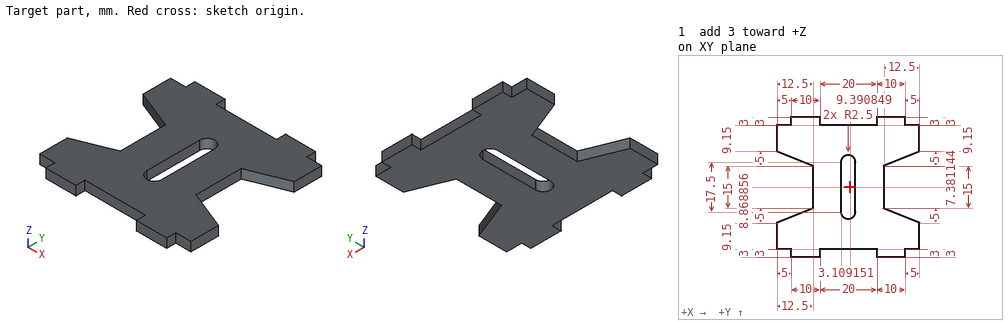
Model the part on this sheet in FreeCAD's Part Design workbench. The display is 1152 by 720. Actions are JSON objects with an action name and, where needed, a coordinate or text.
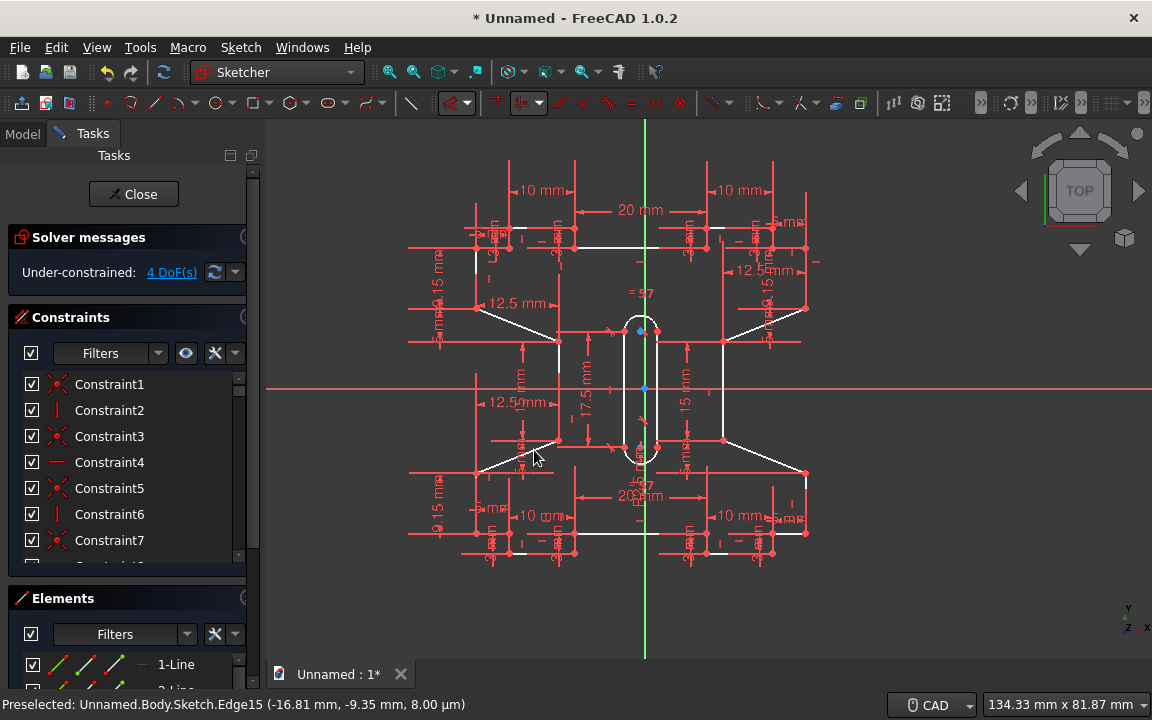
{"action": "left_click", "coordinate": [723, 342]}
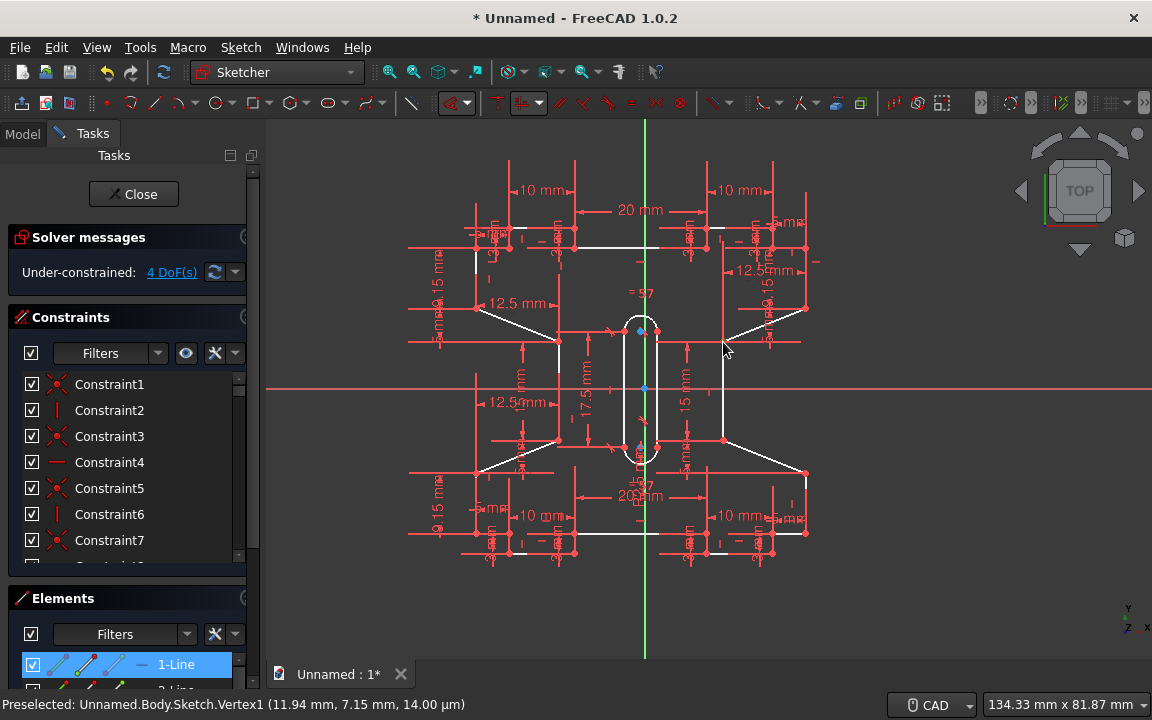
{"action": "left_click", "coordinate": [470, 104]}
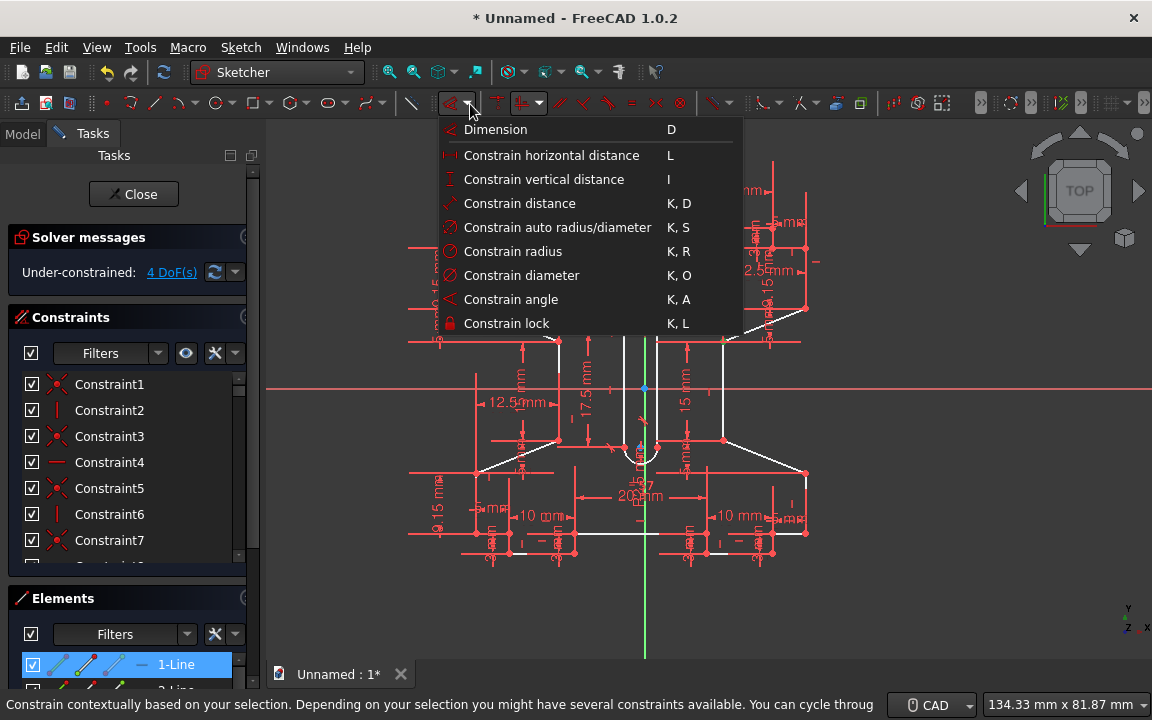
{"action": "left_click", "coordinate": [591, 179]}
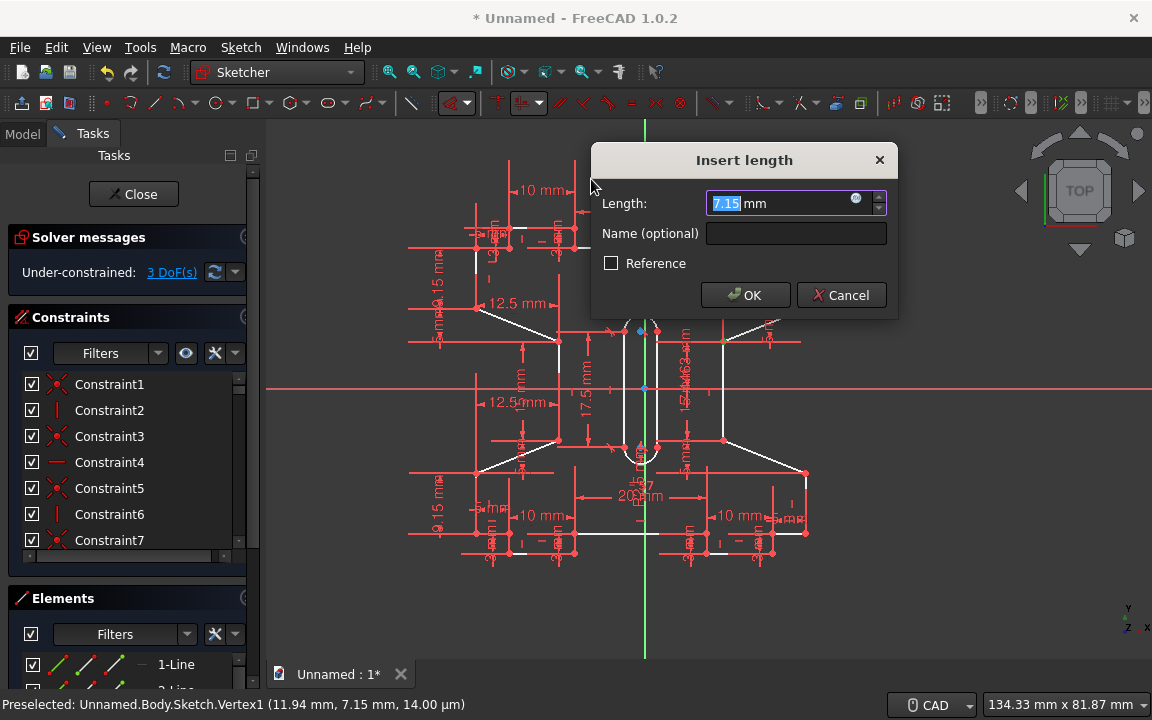
{"action": "type", "text": "7.381144"}
{"action": "key", "text": "Return"}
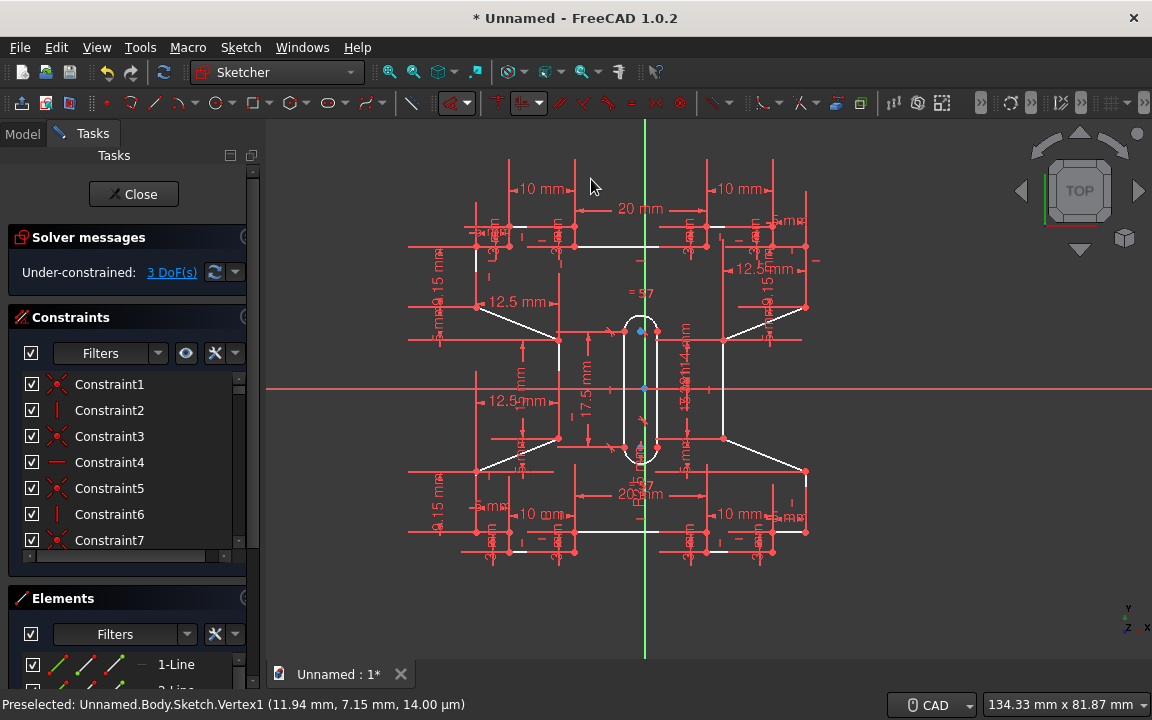
{"action": "left_click", "coordinate": [707, 227]}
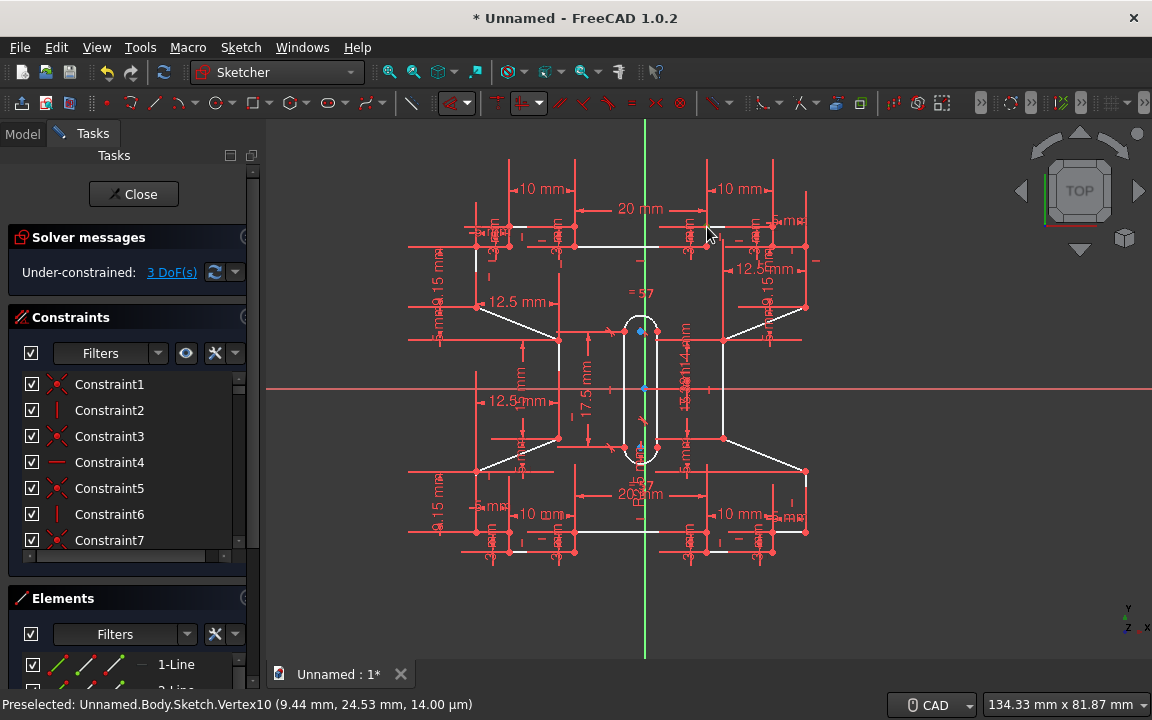
{"action": "key", "text": "l"}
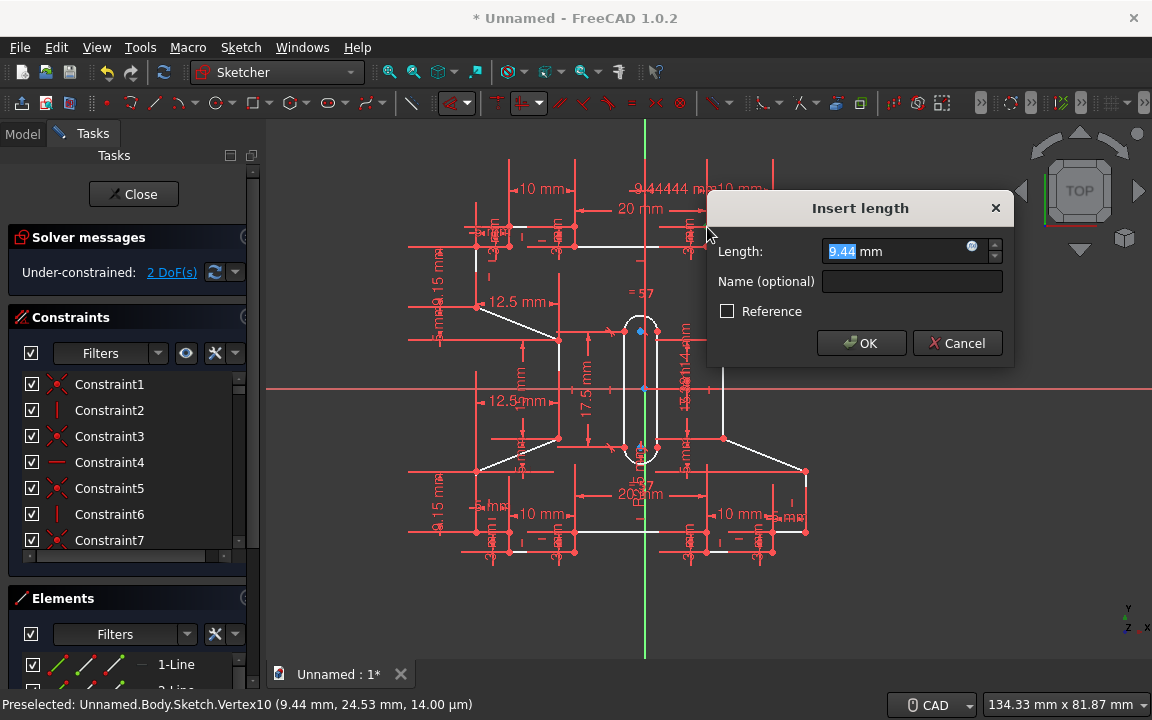
{"action": "type", "text": "9.390849"}
{"action": "key", "text": "Return"}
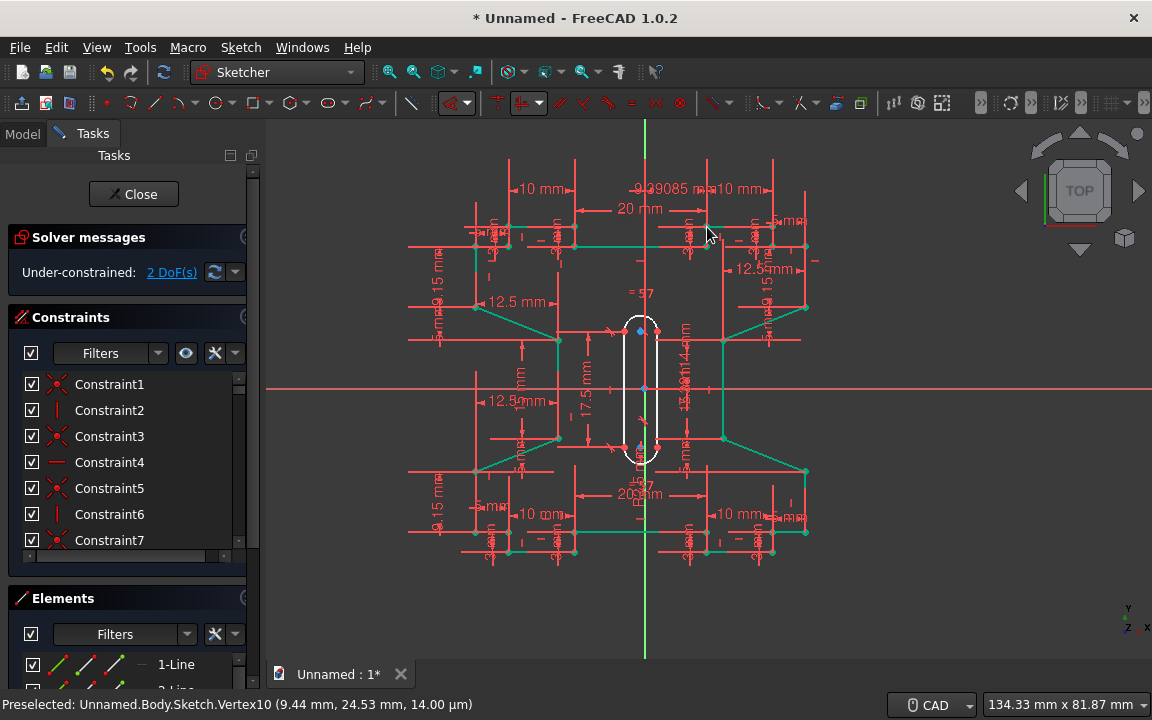
{"action": "scroll", "coordinate": [624, 447], "scroll_direction": "up", "scroll_amount": 4}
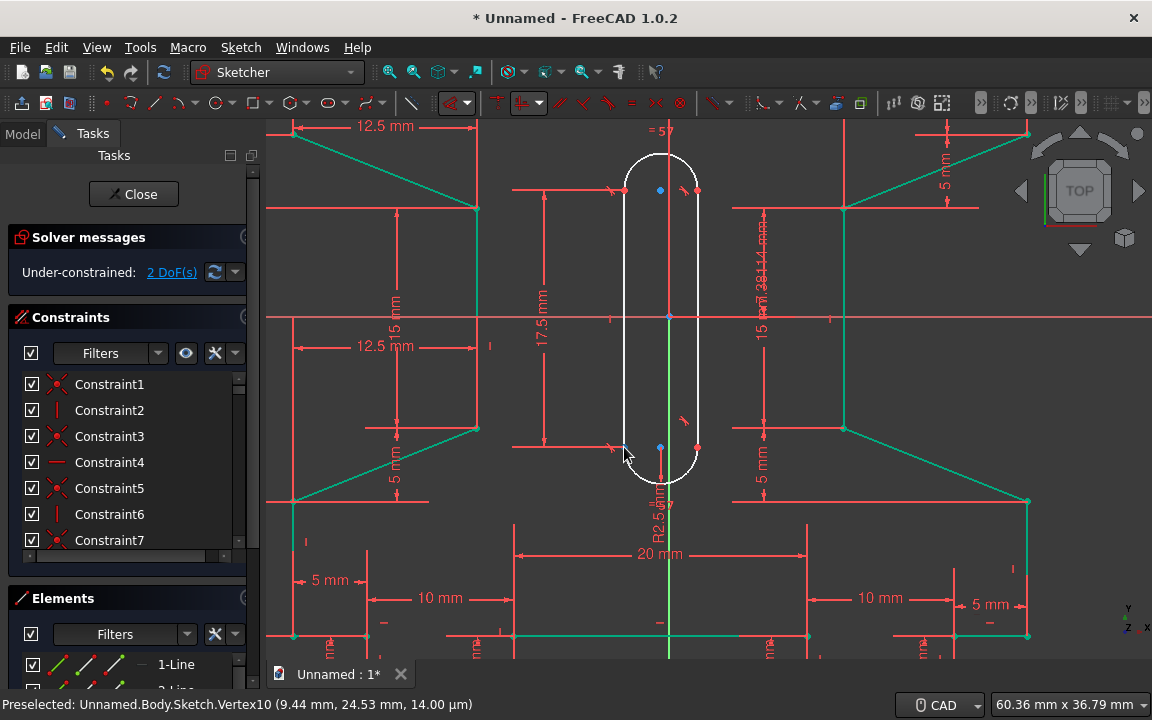
{"action": "left_click", "coordinate": [624, 447]}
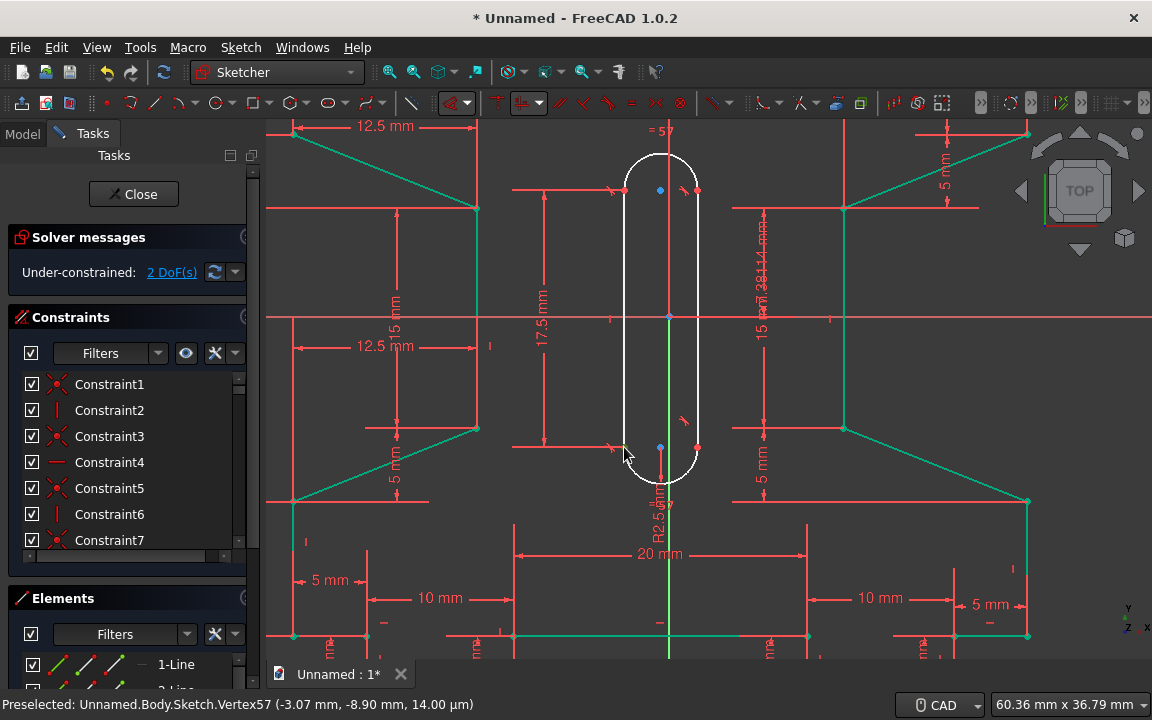
{"action": "left_click", "coordinate": [470, 104]}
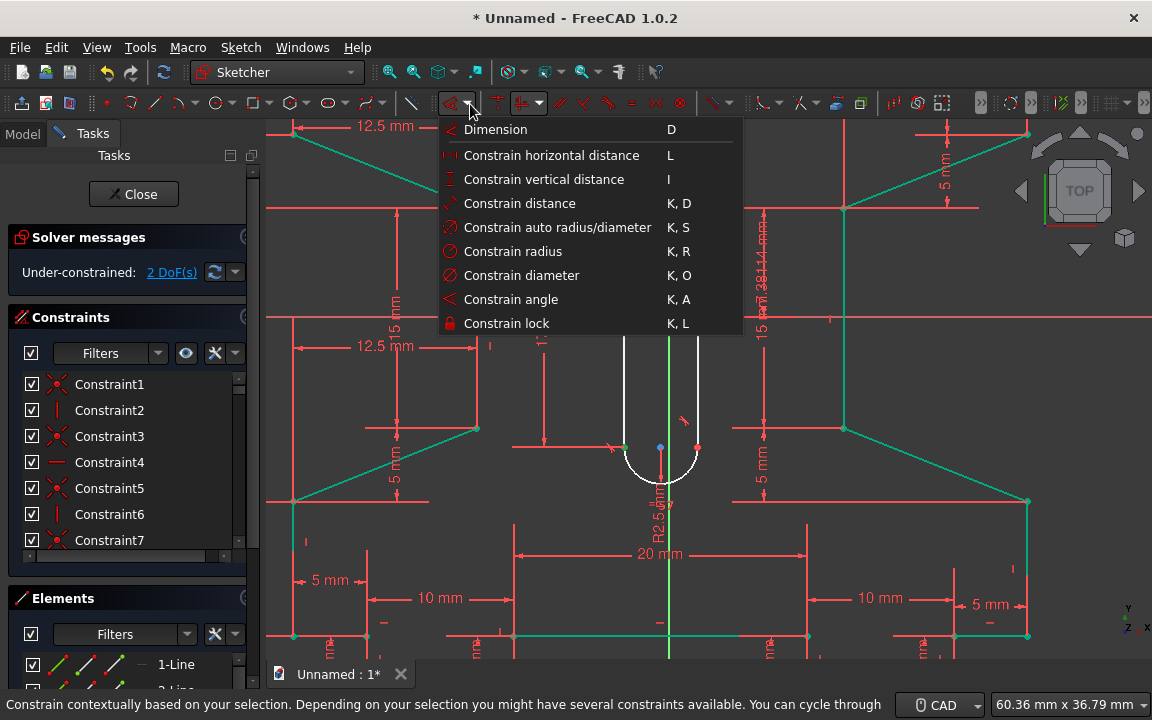
{"action": "left_click", "coordinate": [591, 155]}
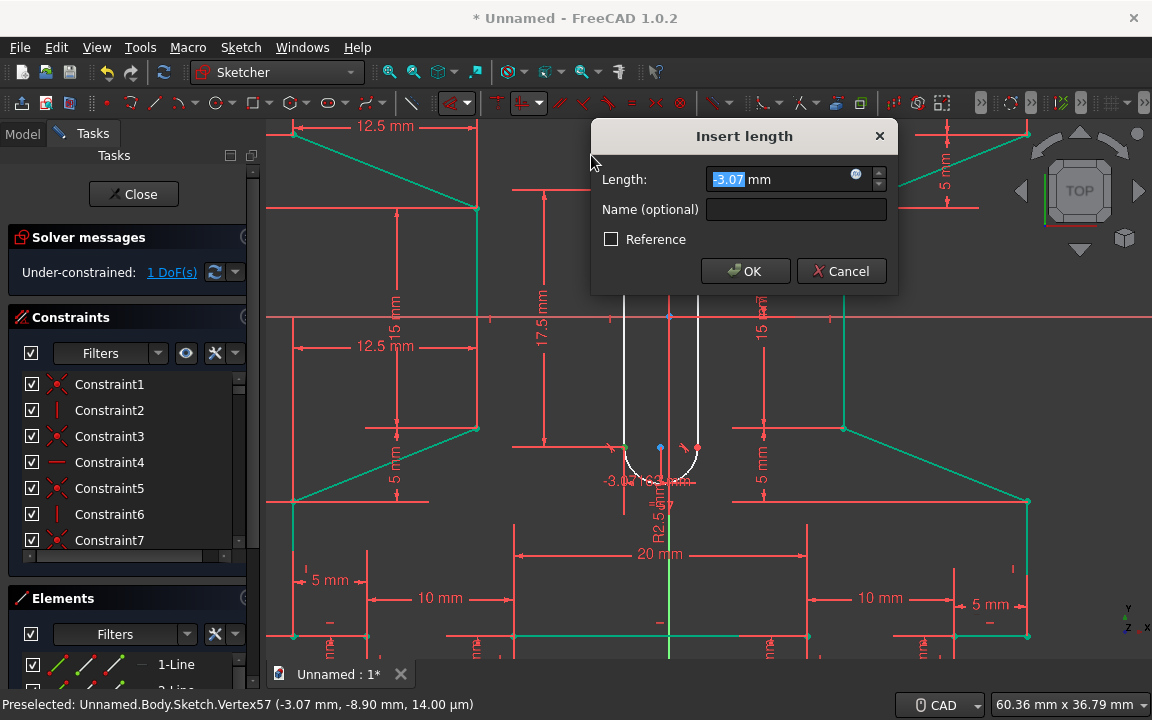
{"action": "type", "text": "-3.109151"}
{"action": "key", "text": "Return"}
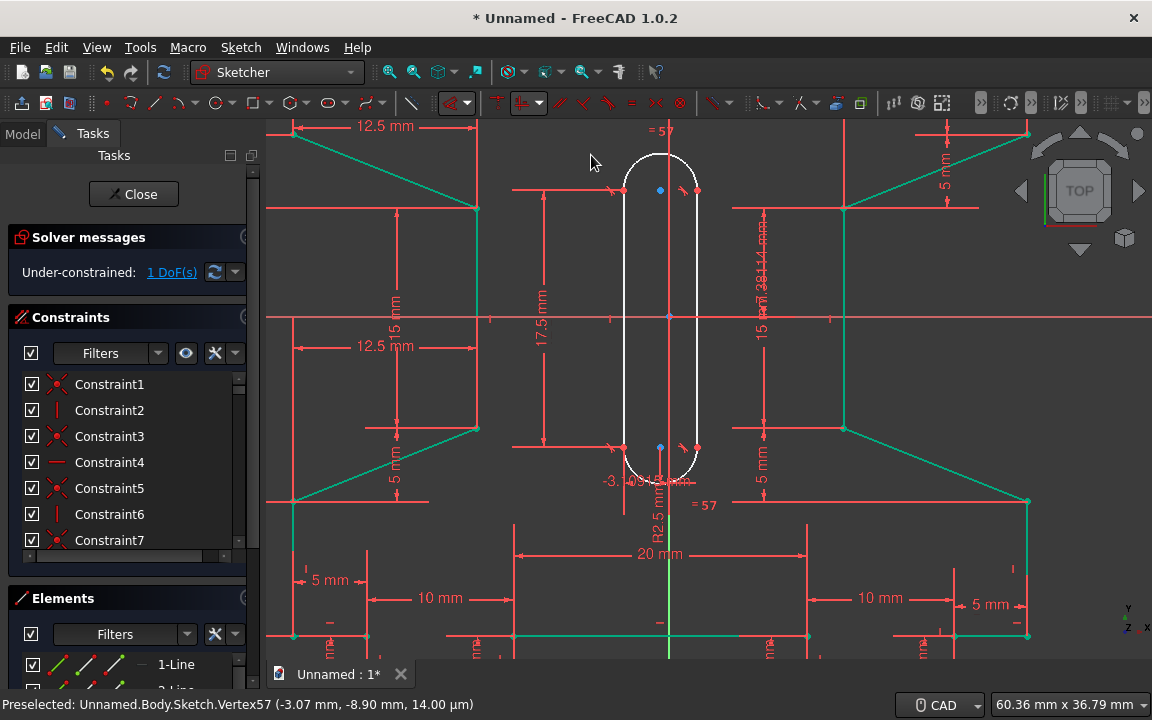
{"action": "left_click", "coordinate": [624, 447]}